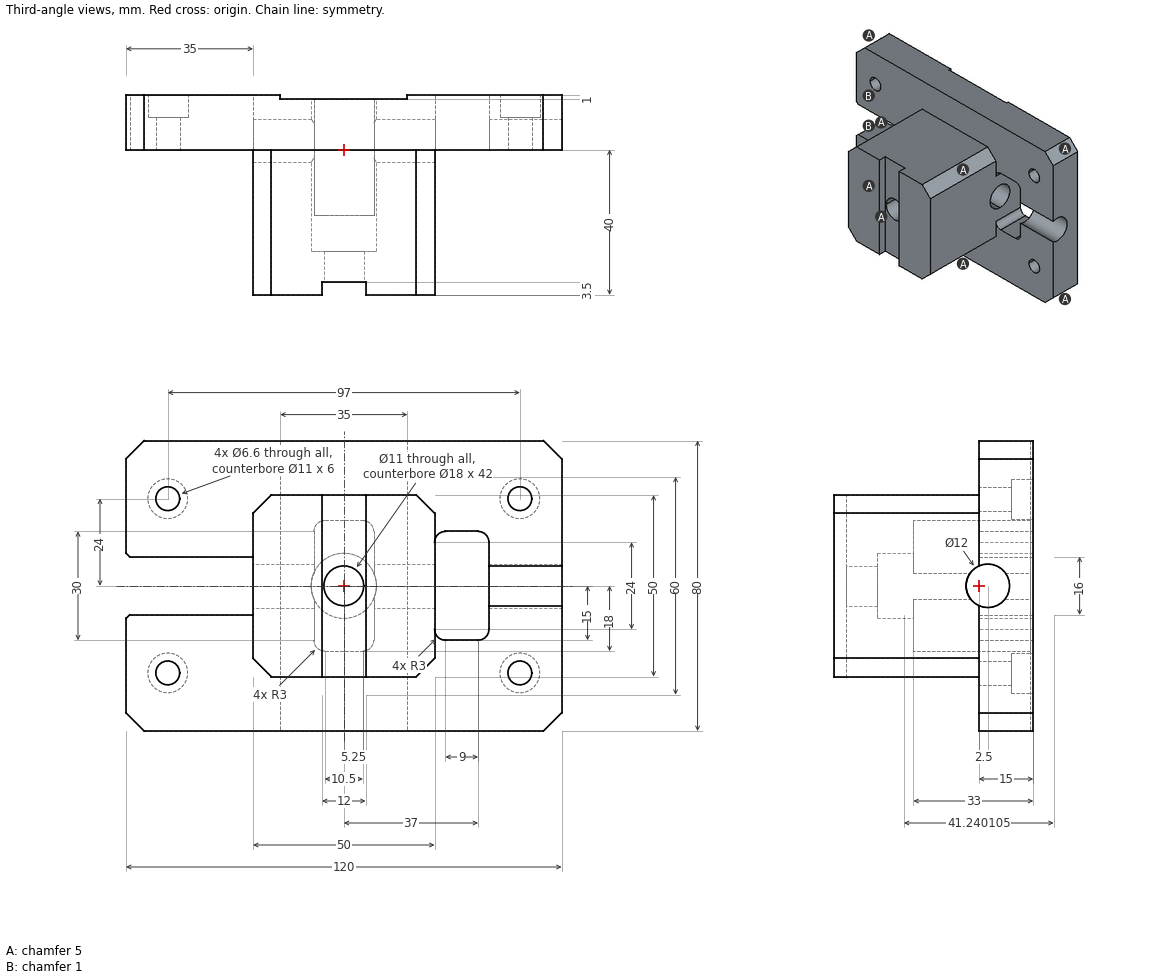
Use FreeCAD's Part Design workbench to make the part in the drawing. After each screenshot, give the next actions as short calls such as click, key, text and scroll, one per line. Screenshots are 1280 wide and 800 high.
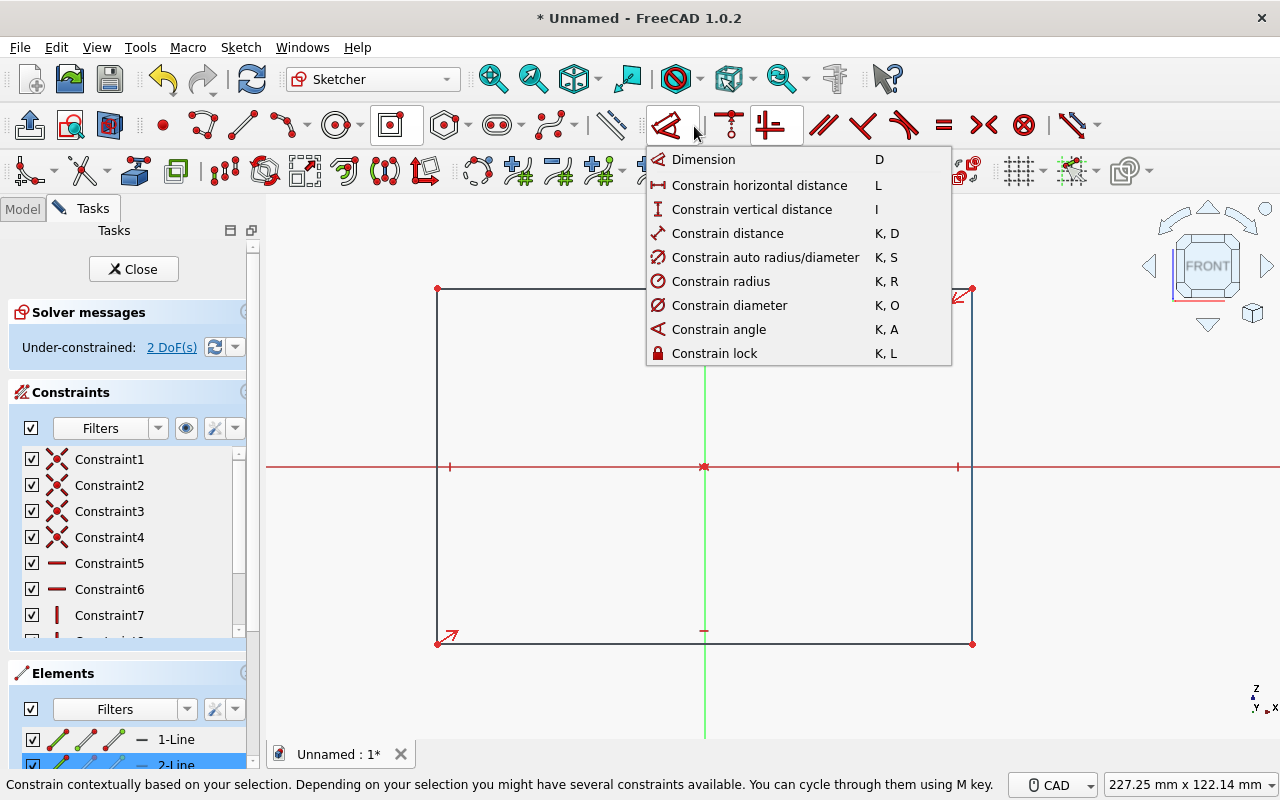
click(799, 209)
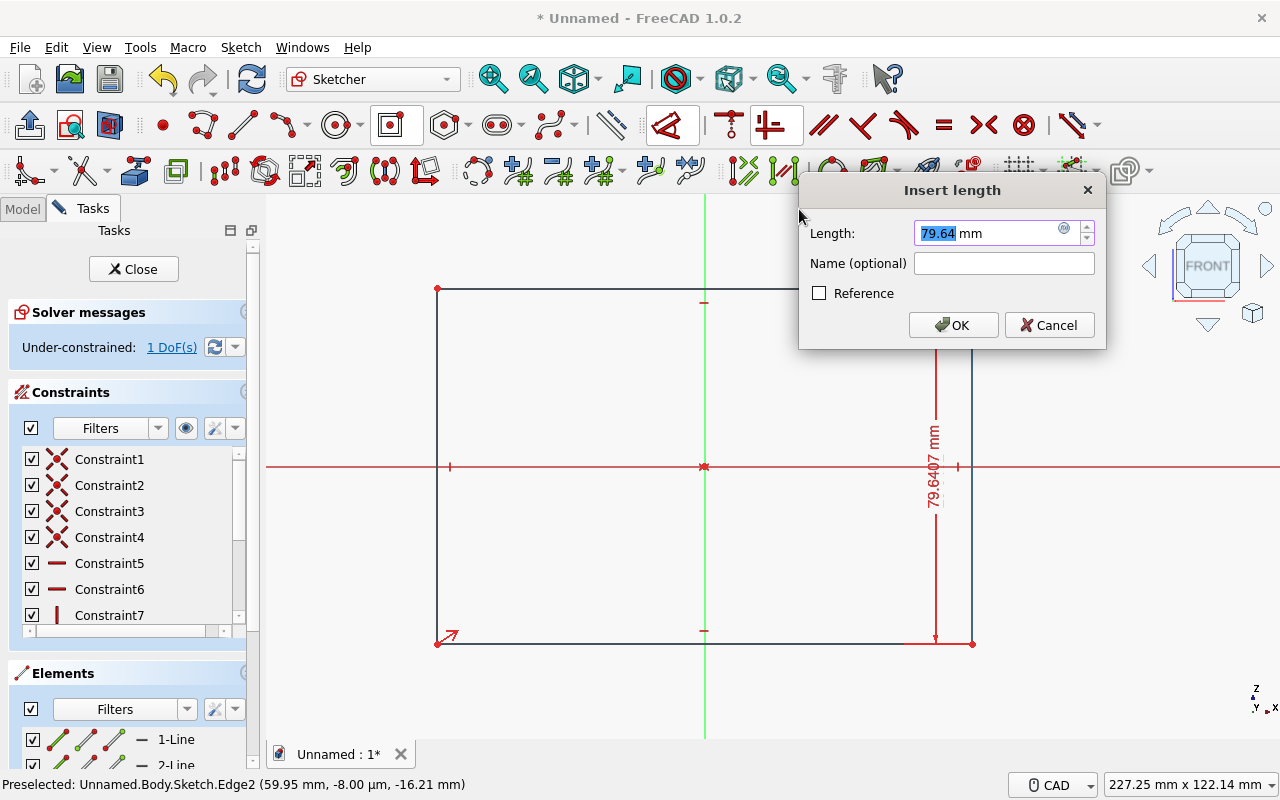
text(80)
key(Return)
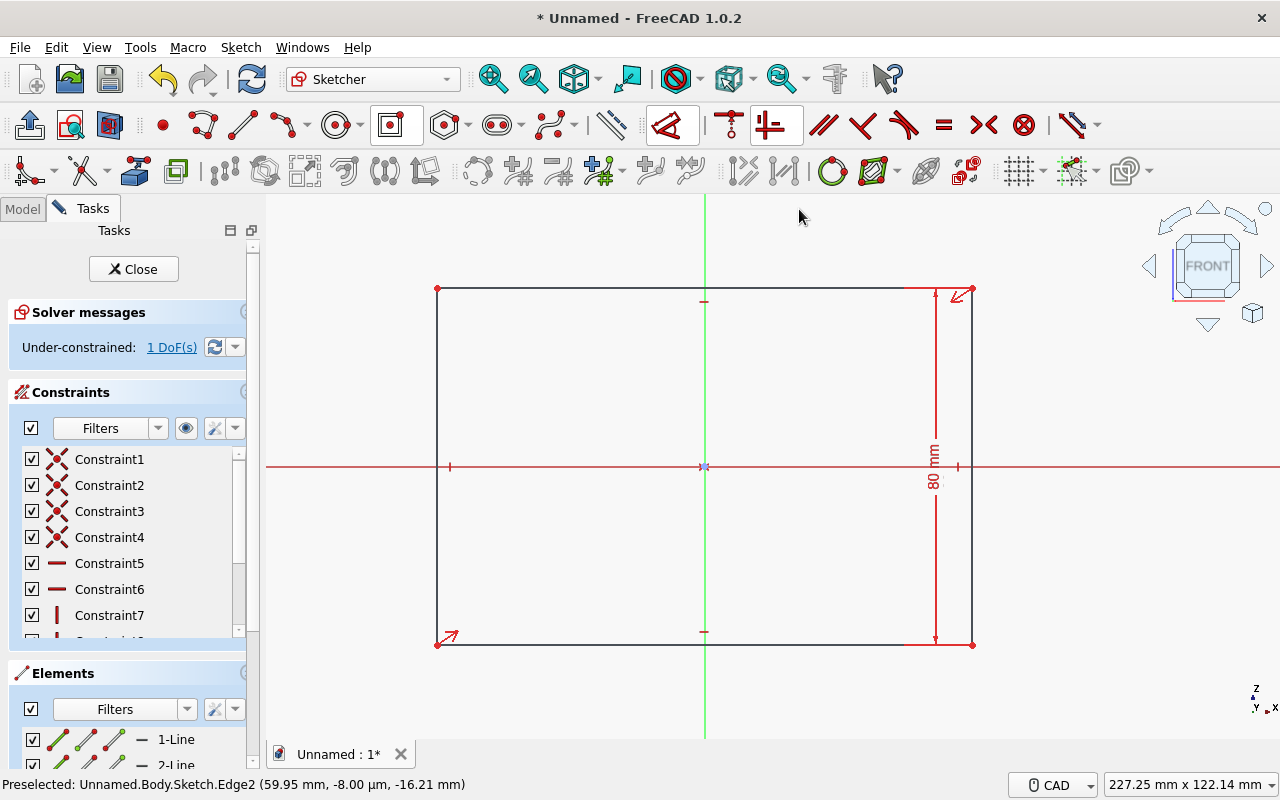
click(598, 645)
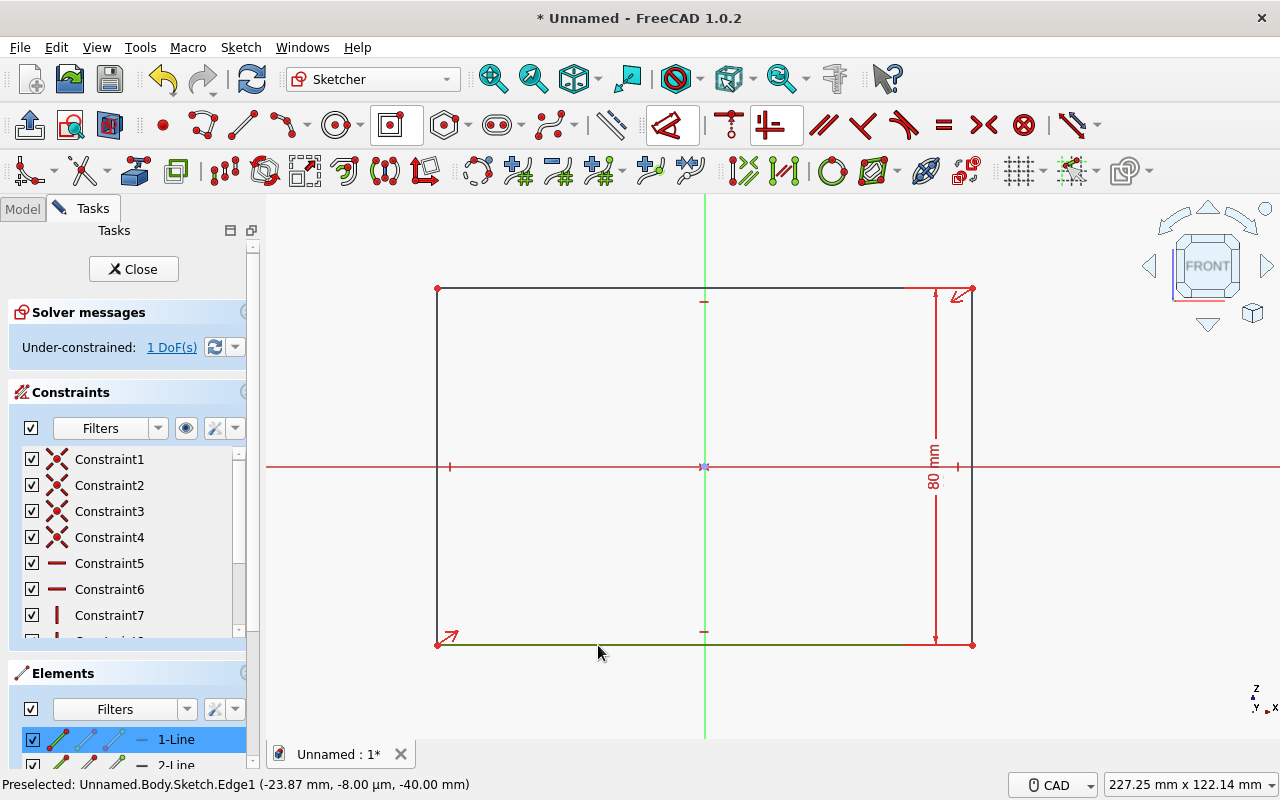
click(694, 126)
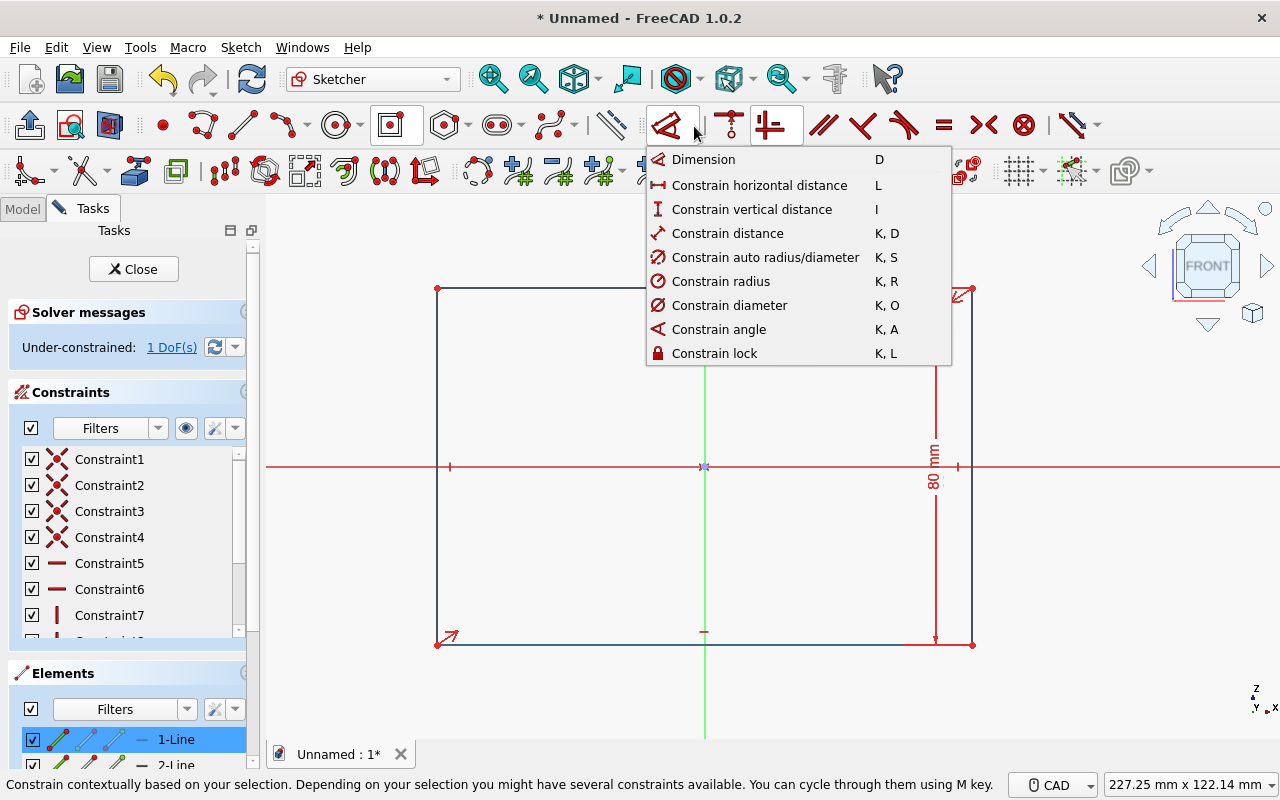
click(799, 185)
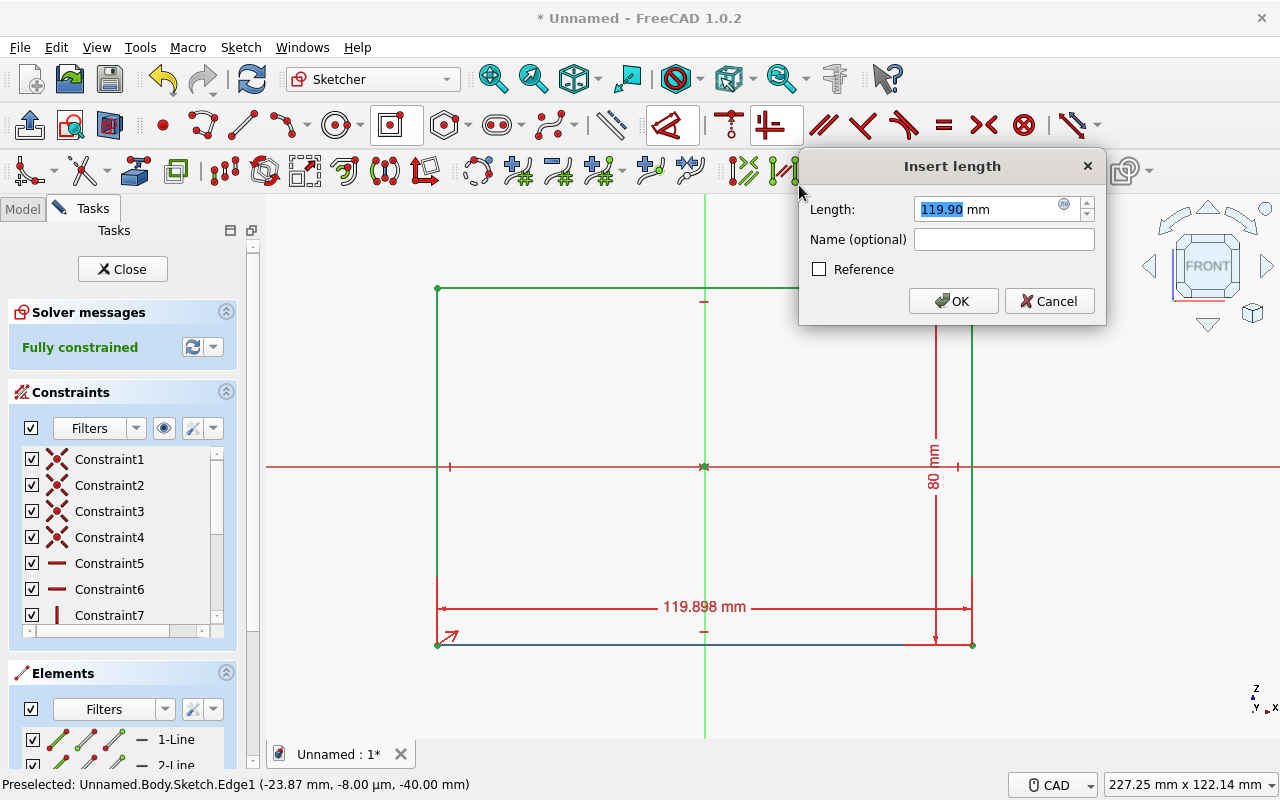
text(120)
key(Return)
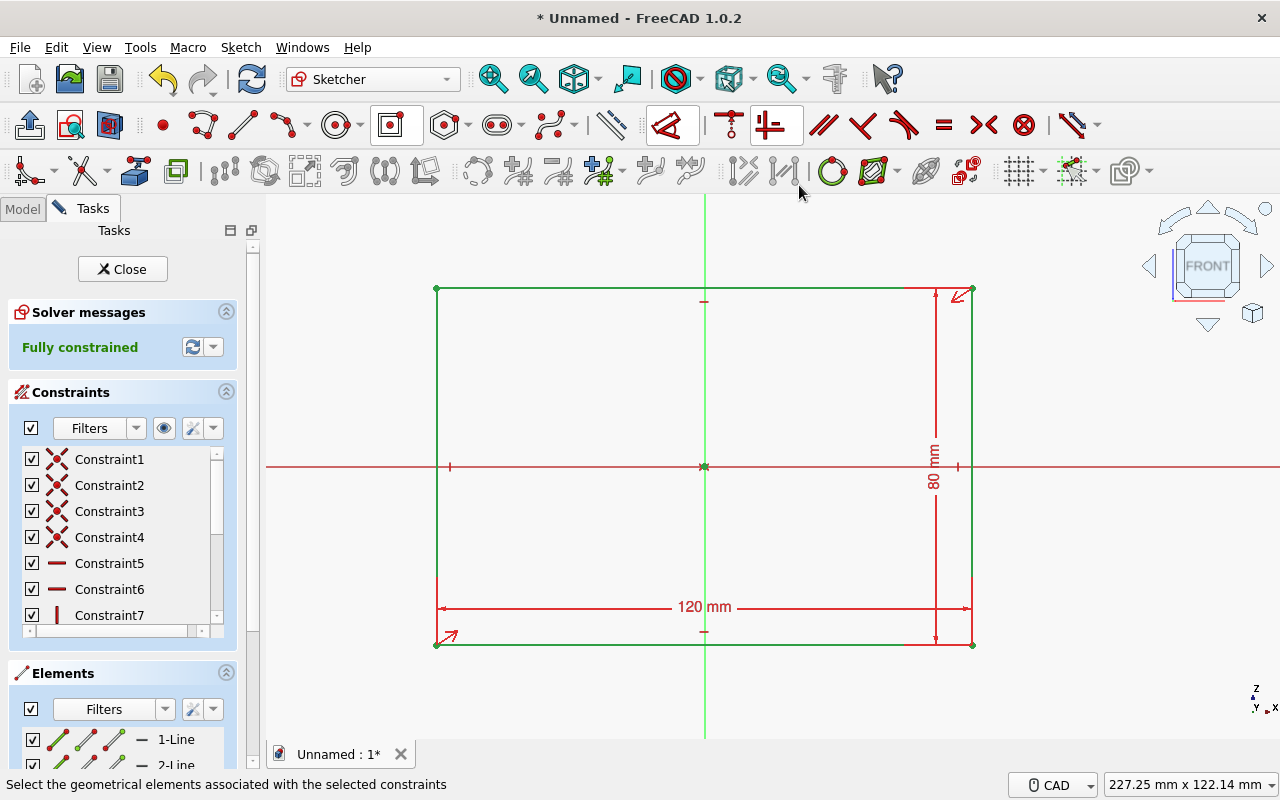
click(123, 269)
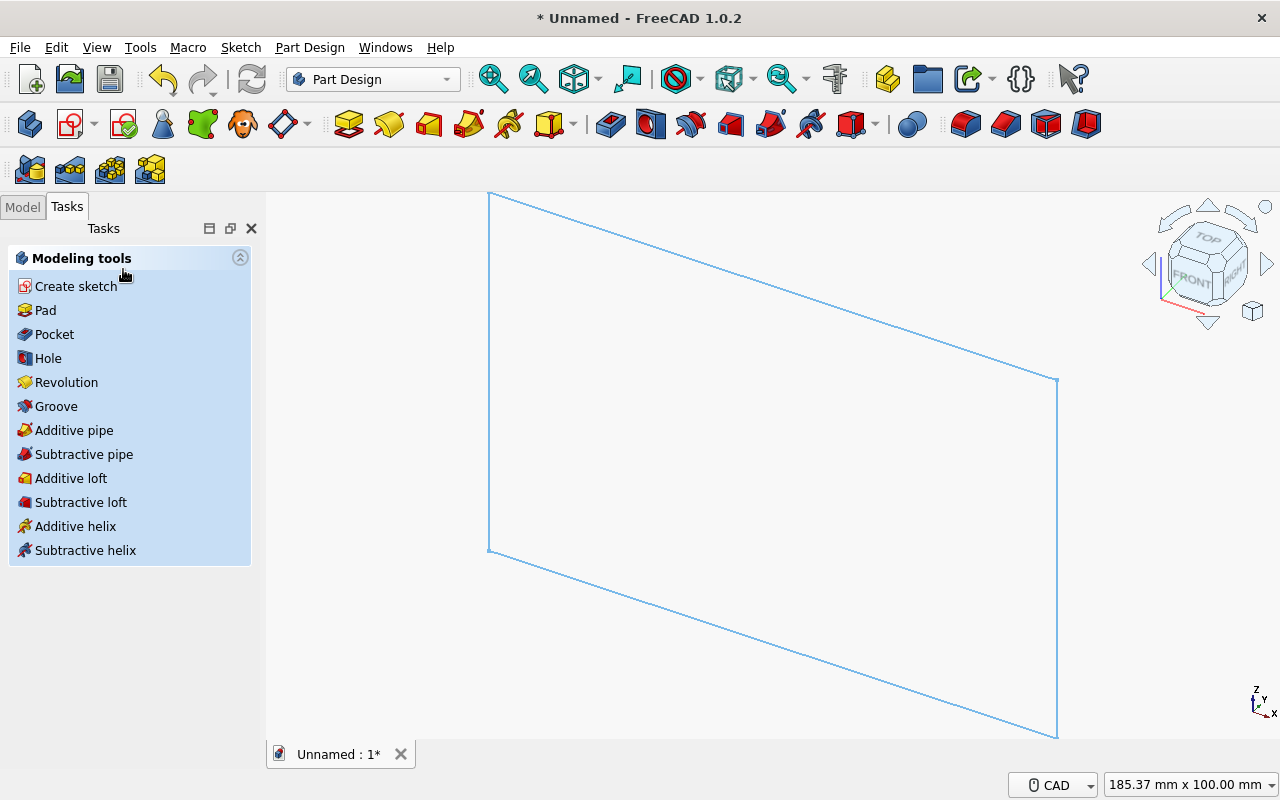
click(350, 124)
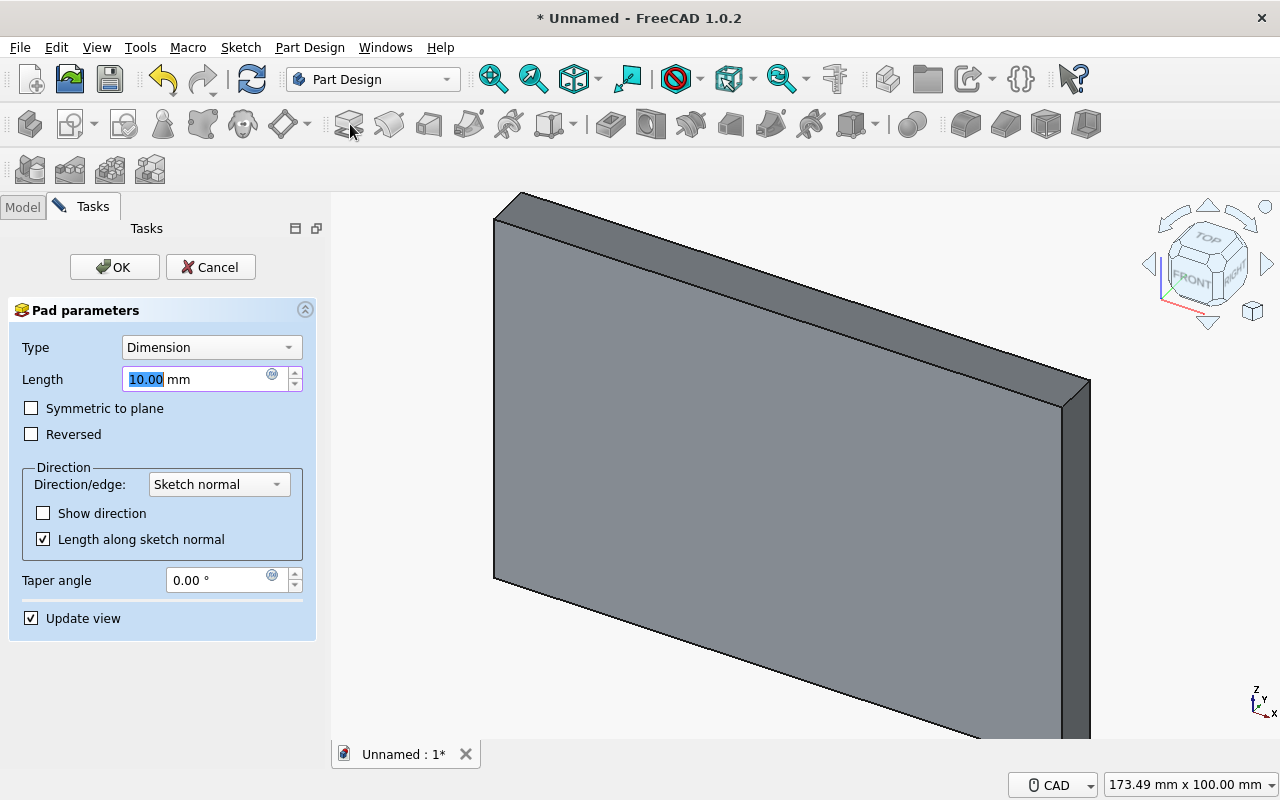
text(15)
key(Tab)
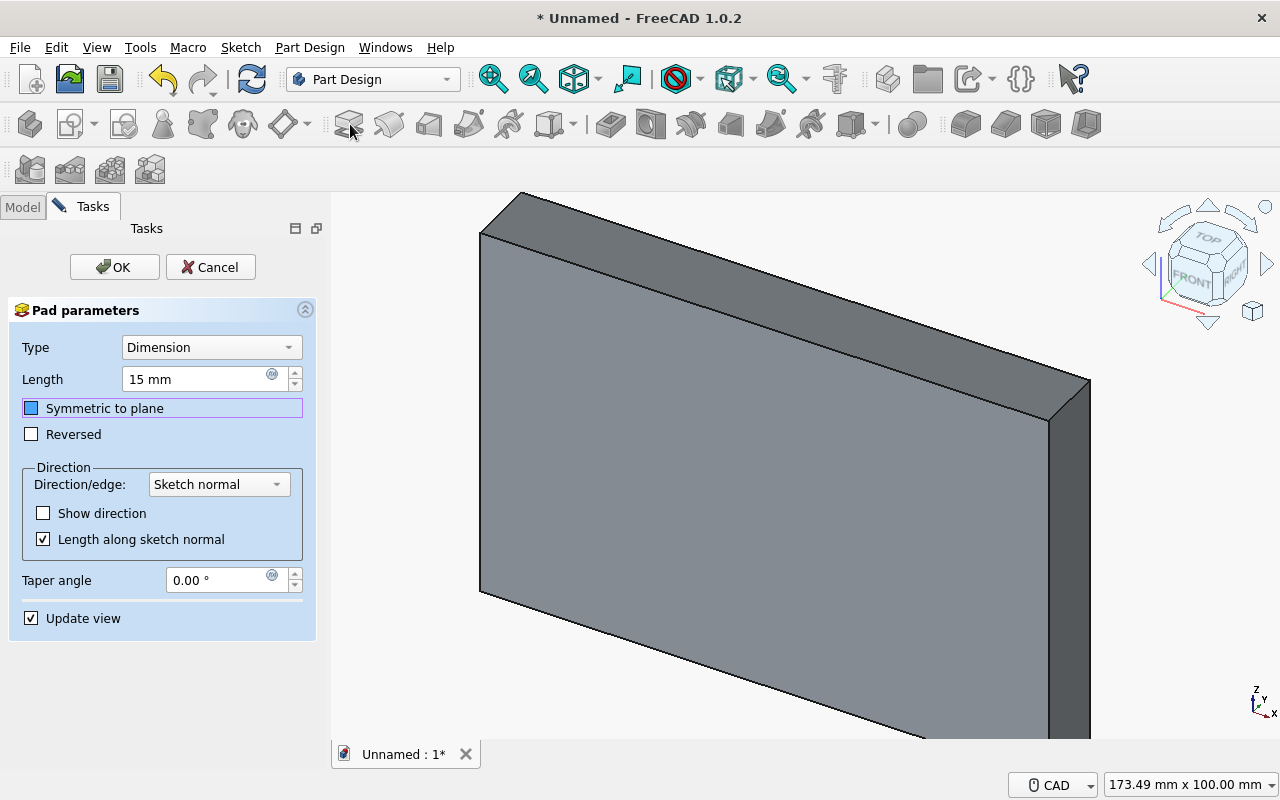
click(30, 434)